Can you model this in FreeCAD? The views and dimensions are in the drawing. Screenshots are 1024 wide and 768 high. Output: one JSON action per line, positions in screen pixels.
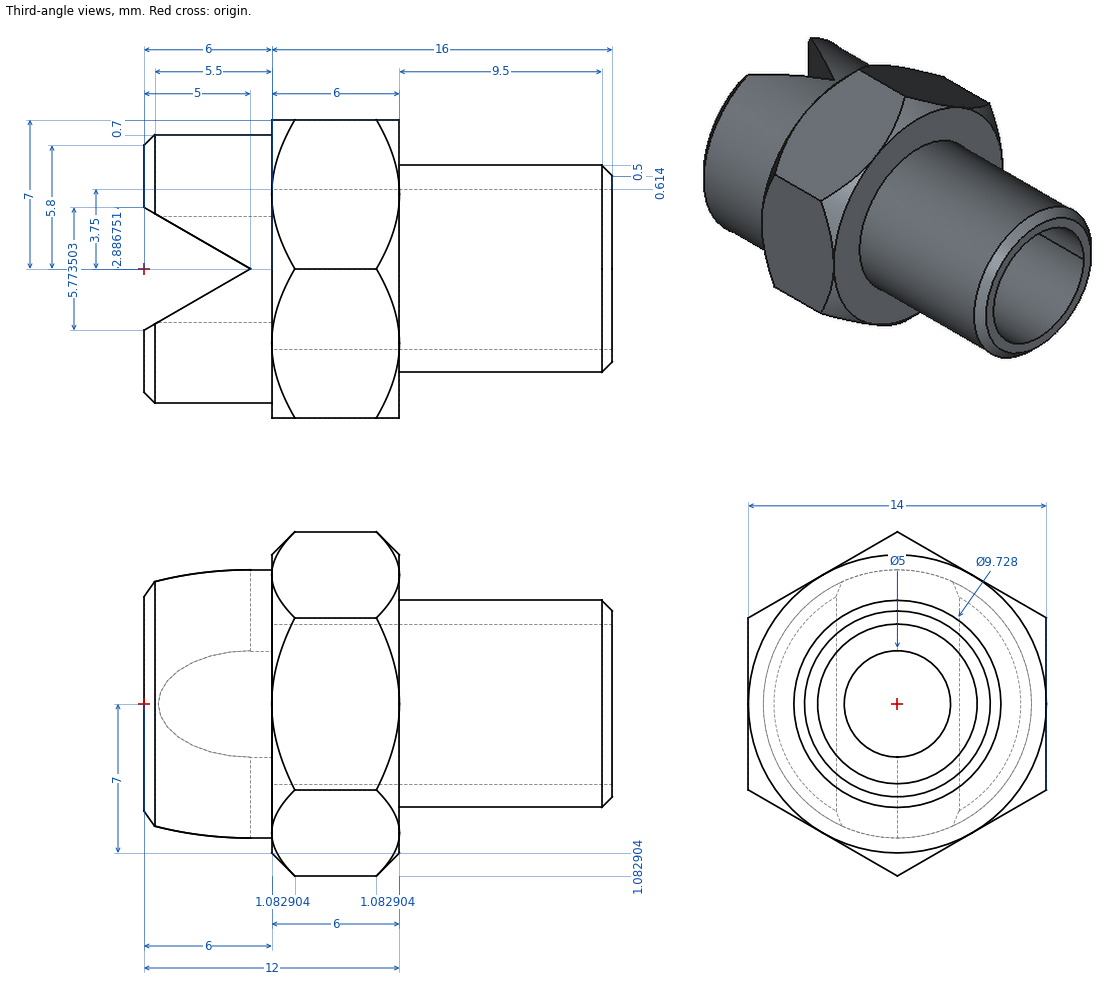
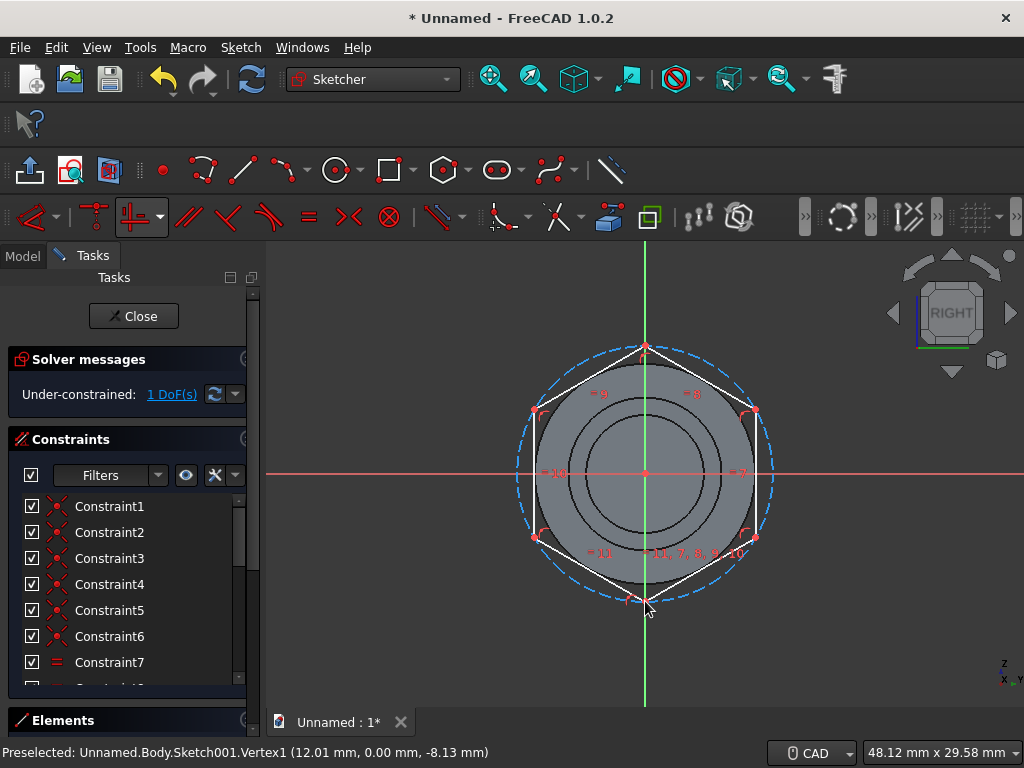
{"action": "left_click", "coordinate": [336, 170]}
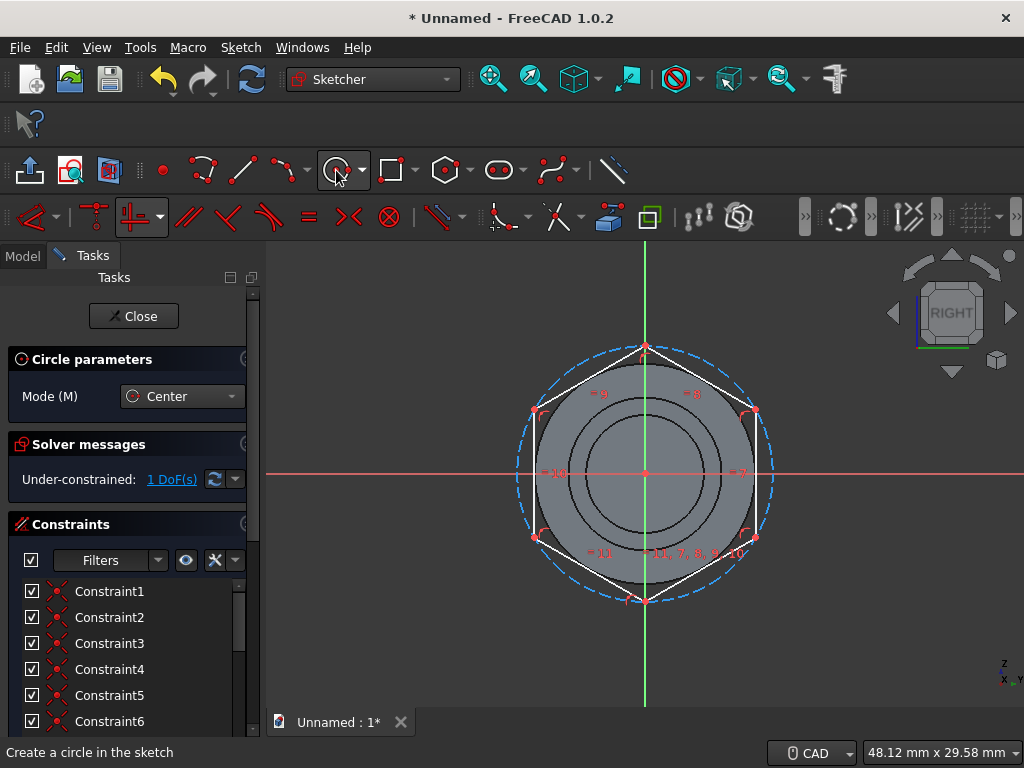
{"action": "left_click", "coordinate": [645, 474]}
{"action": "left_click", "coordinate": [699, 420]}
{"action": "key", "text": "Escape"}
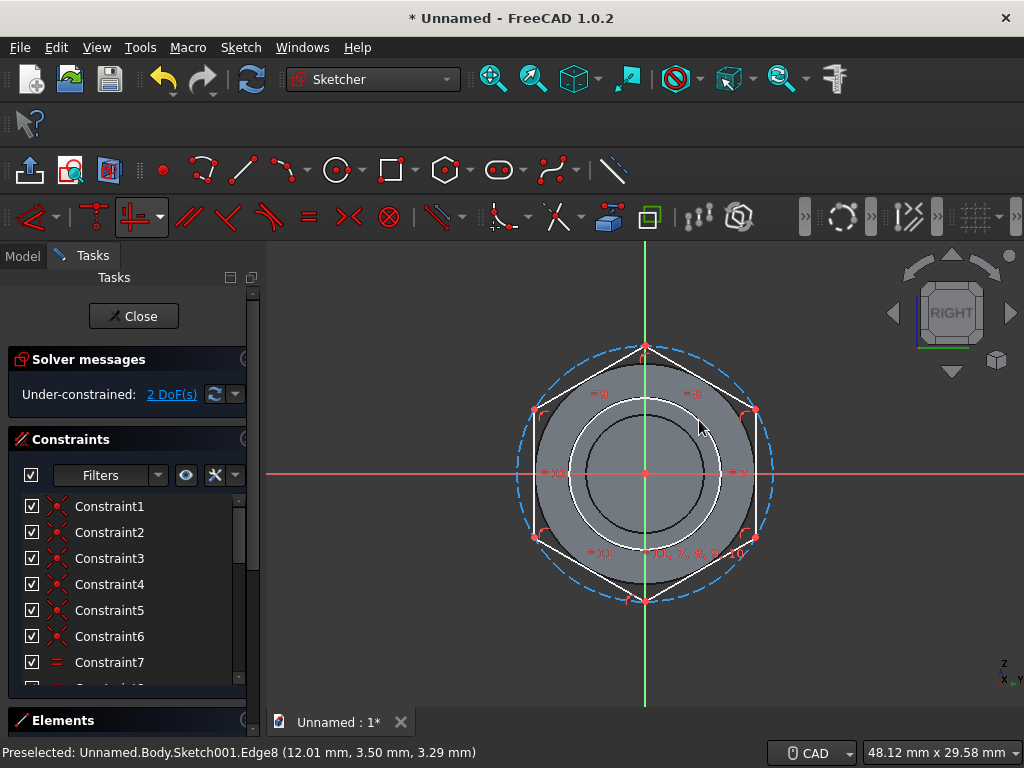
{"action": "left_click", "coordinate": [32, 218]}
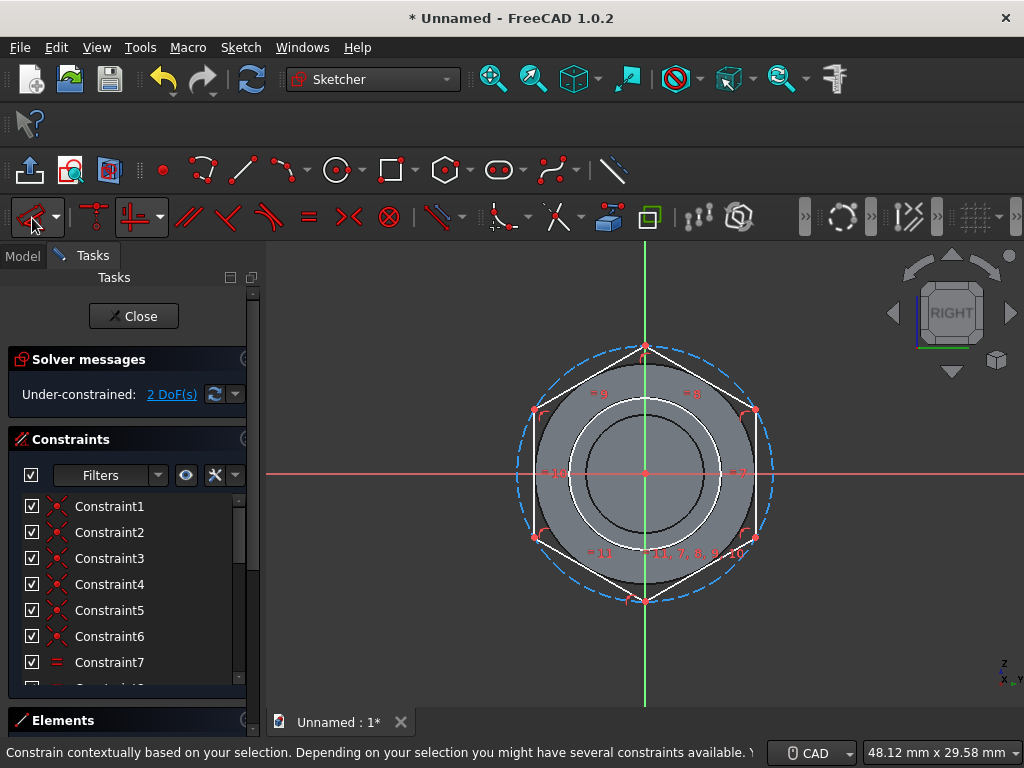
{"action": "left_click", "coordinate": [698, 420]}
{"action": "left_click", "coordinate": [754, 363]}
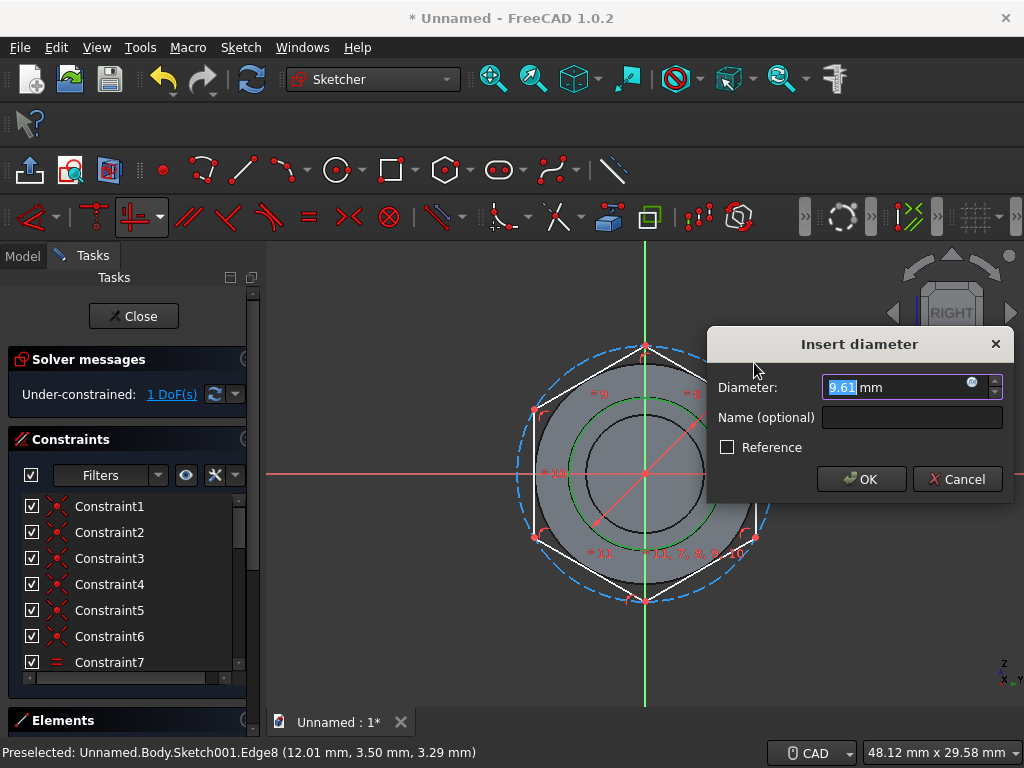
{"action": "type", "text": "9.728"}
{"action": "key", "text": "Return"}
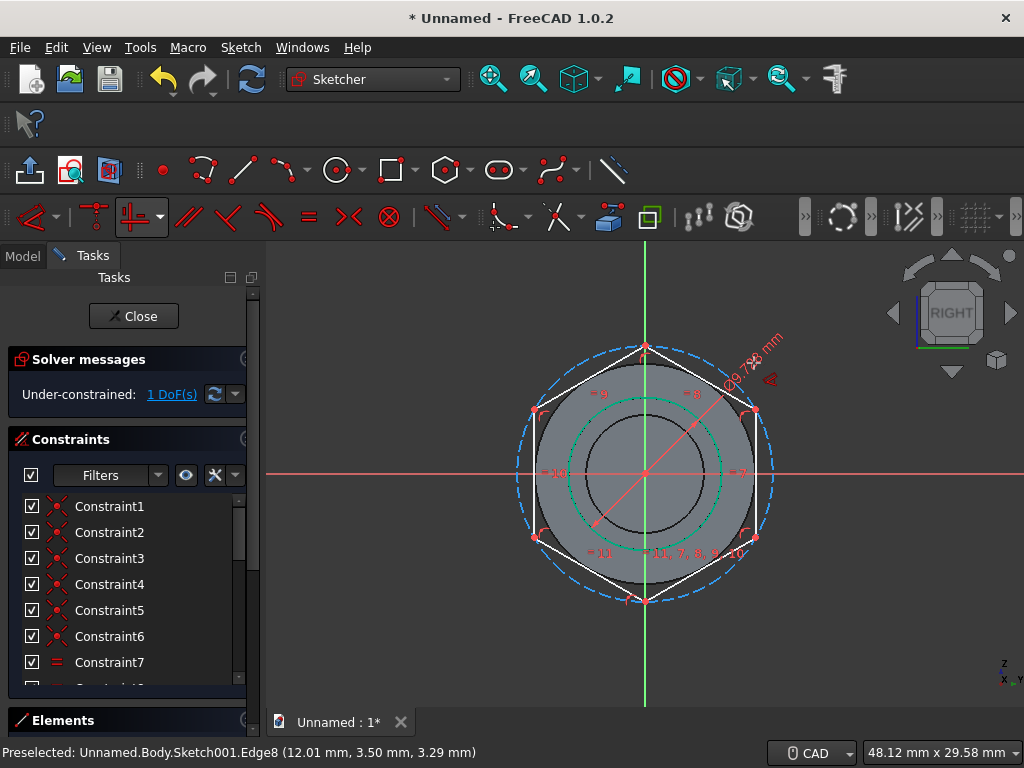
{"action": "left_click", "coordinate": [534, 410]}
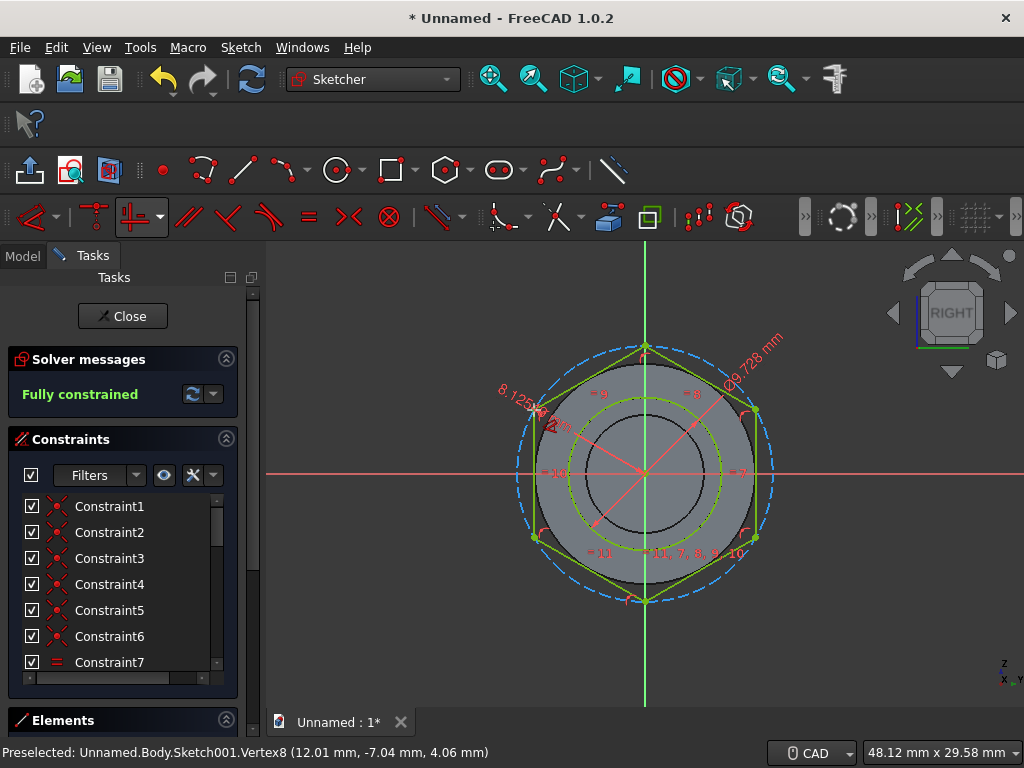
{"action": "left_click", "coordinate": [756, 538]}
{"action": "left_click", "coordinate": [567, 596]}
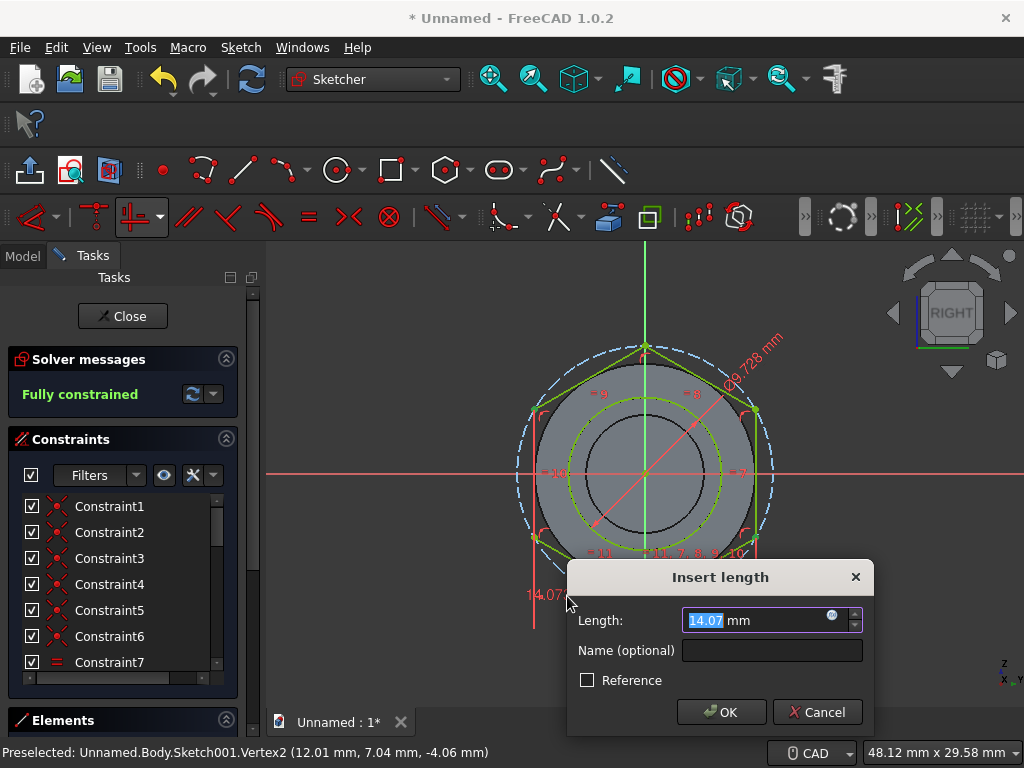
{"action": "type", "text": "14"}
{"action": "key", "text": "Return"}
{"action": "key", "text": "Escape"}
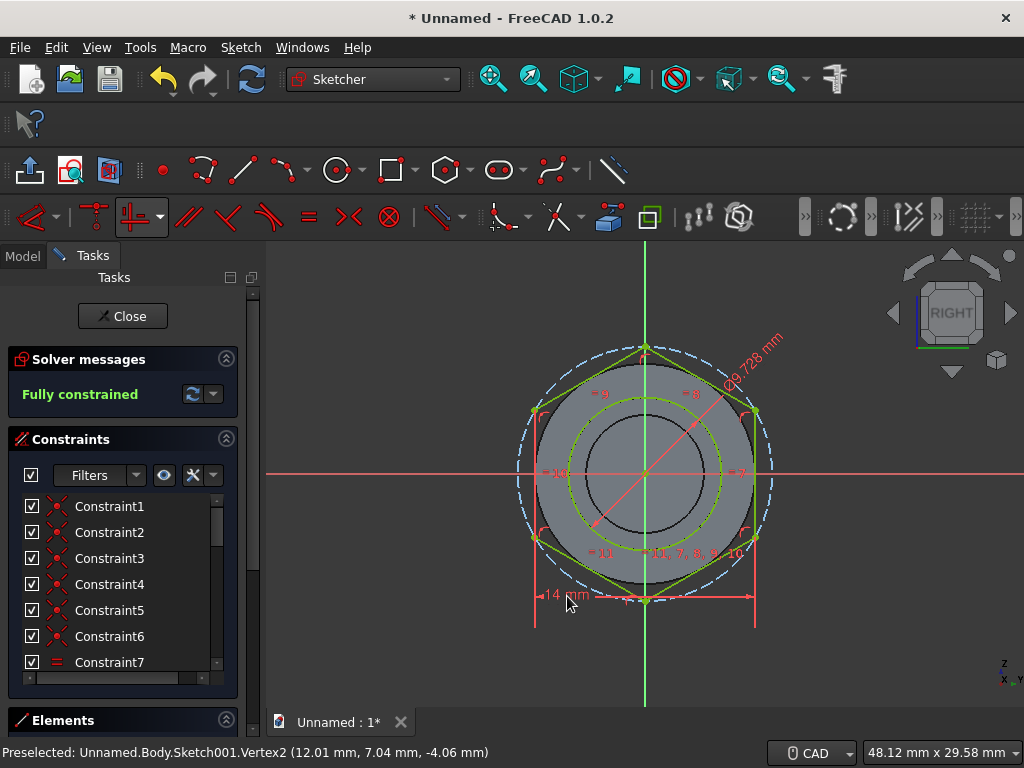
{"action": "left_click", "coordinate": [123, 316]}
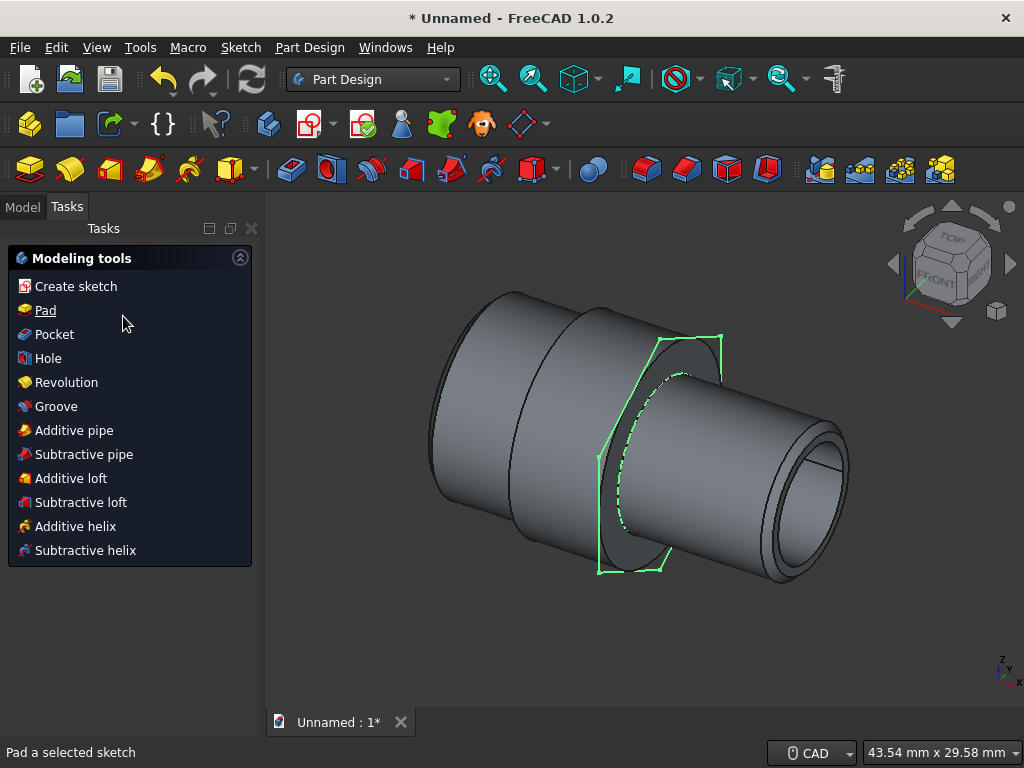
{"action": "left_click", "coordinate": [30, 170]}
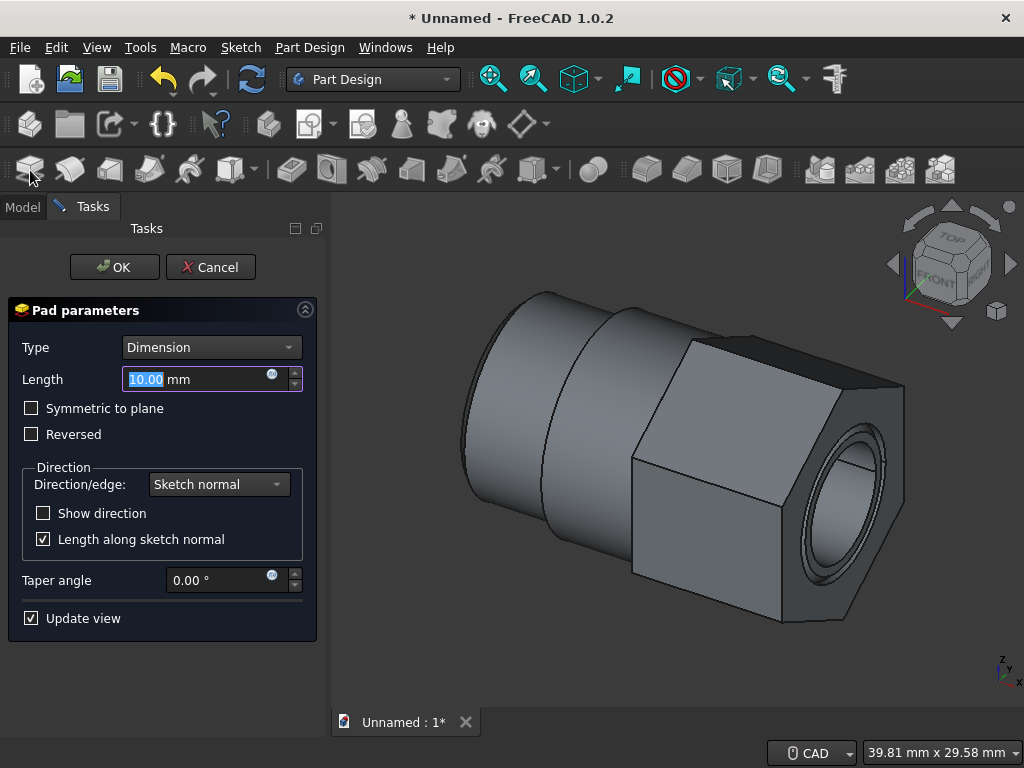
{"action": "type", "text": "6"}
{"action": "key", "text": "Tab"}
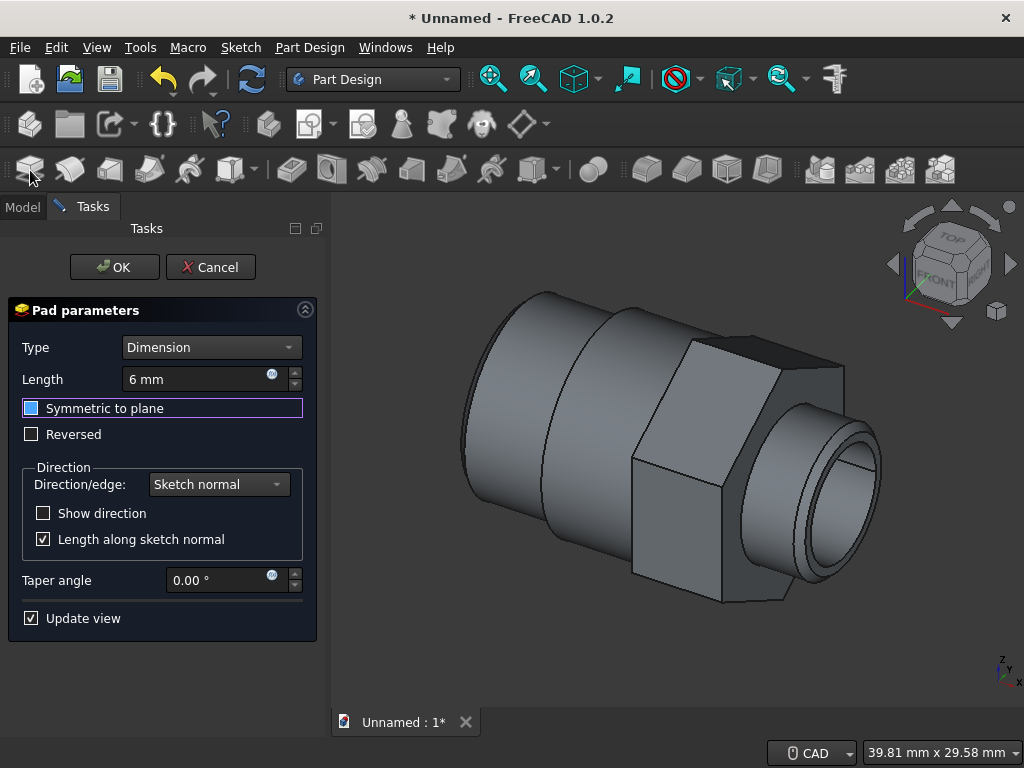
{"action": "left_click", "coordinate": [30, 434]}